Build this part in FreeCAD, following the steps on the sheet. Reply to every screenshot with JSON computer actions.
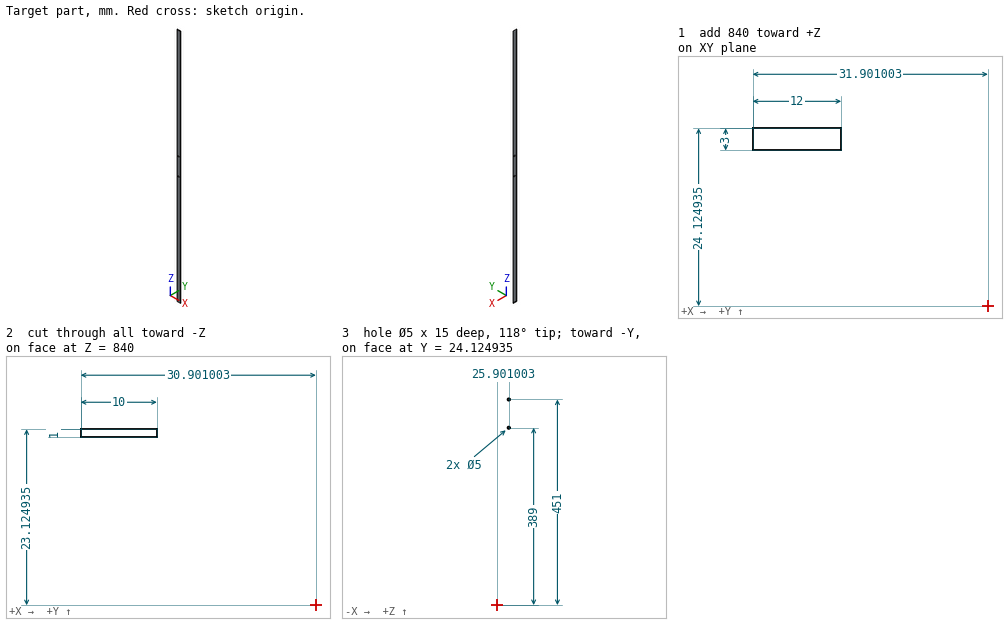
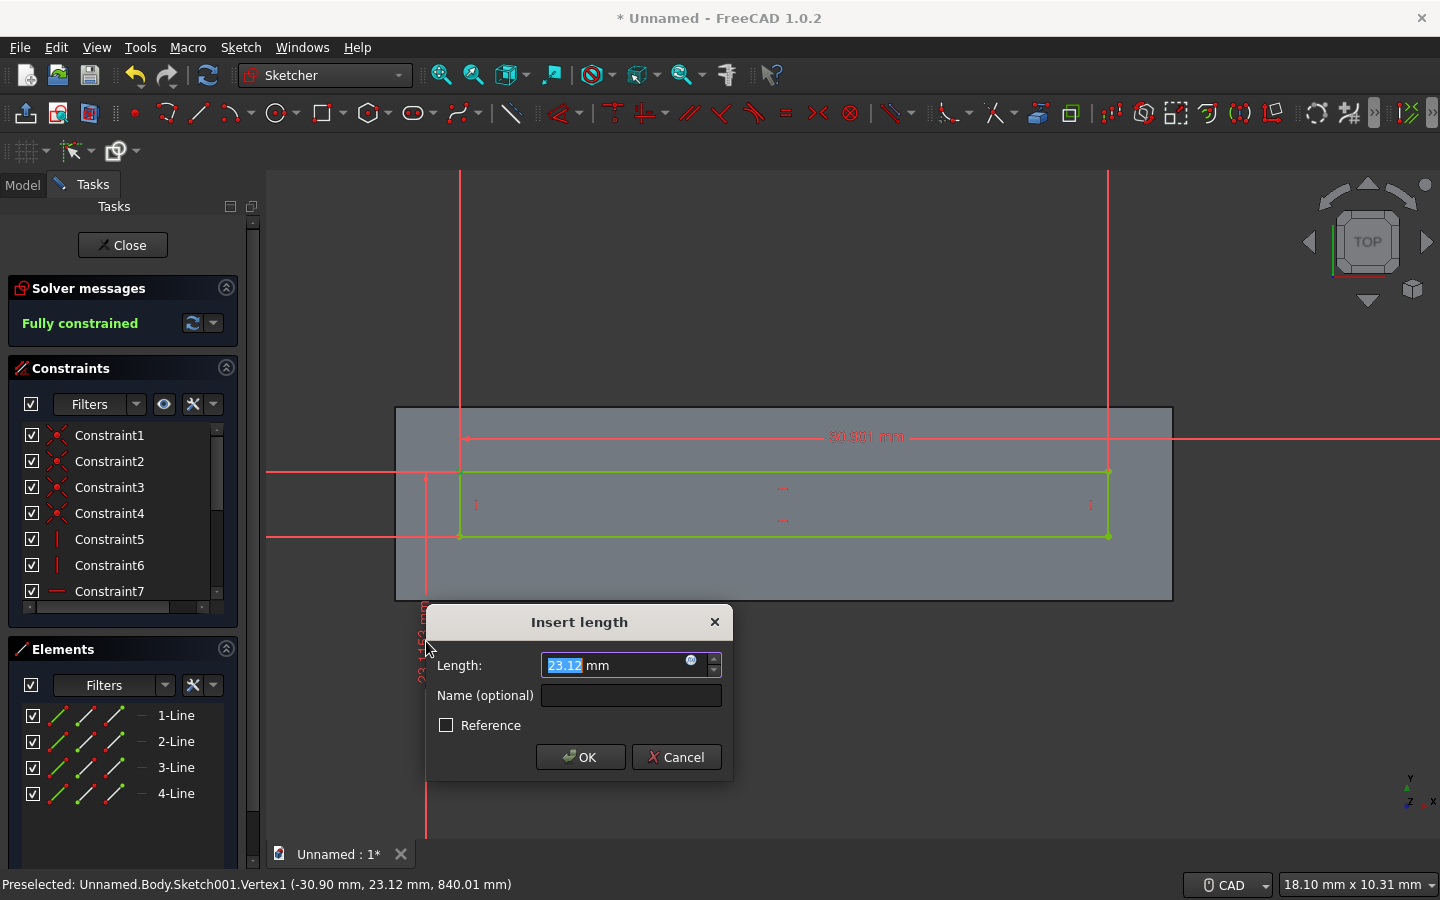
{"action": "type", "text": "23.124935"}
{"action": "key", "text": "Return"}
{"action": "key", "text": "Escape"}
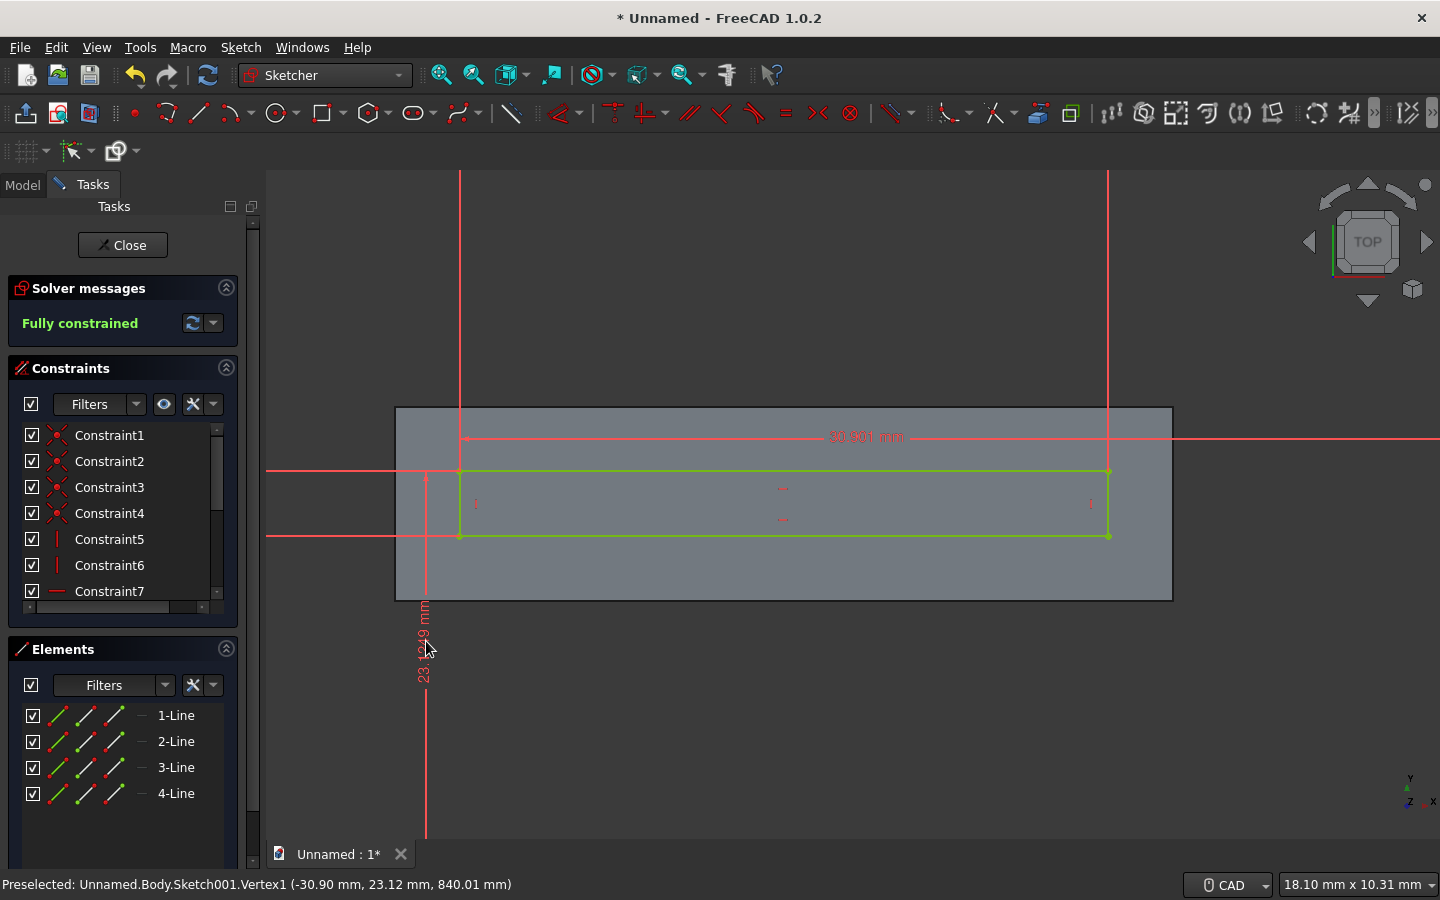
{"action": "left_click", "coordinate": [123, 245]}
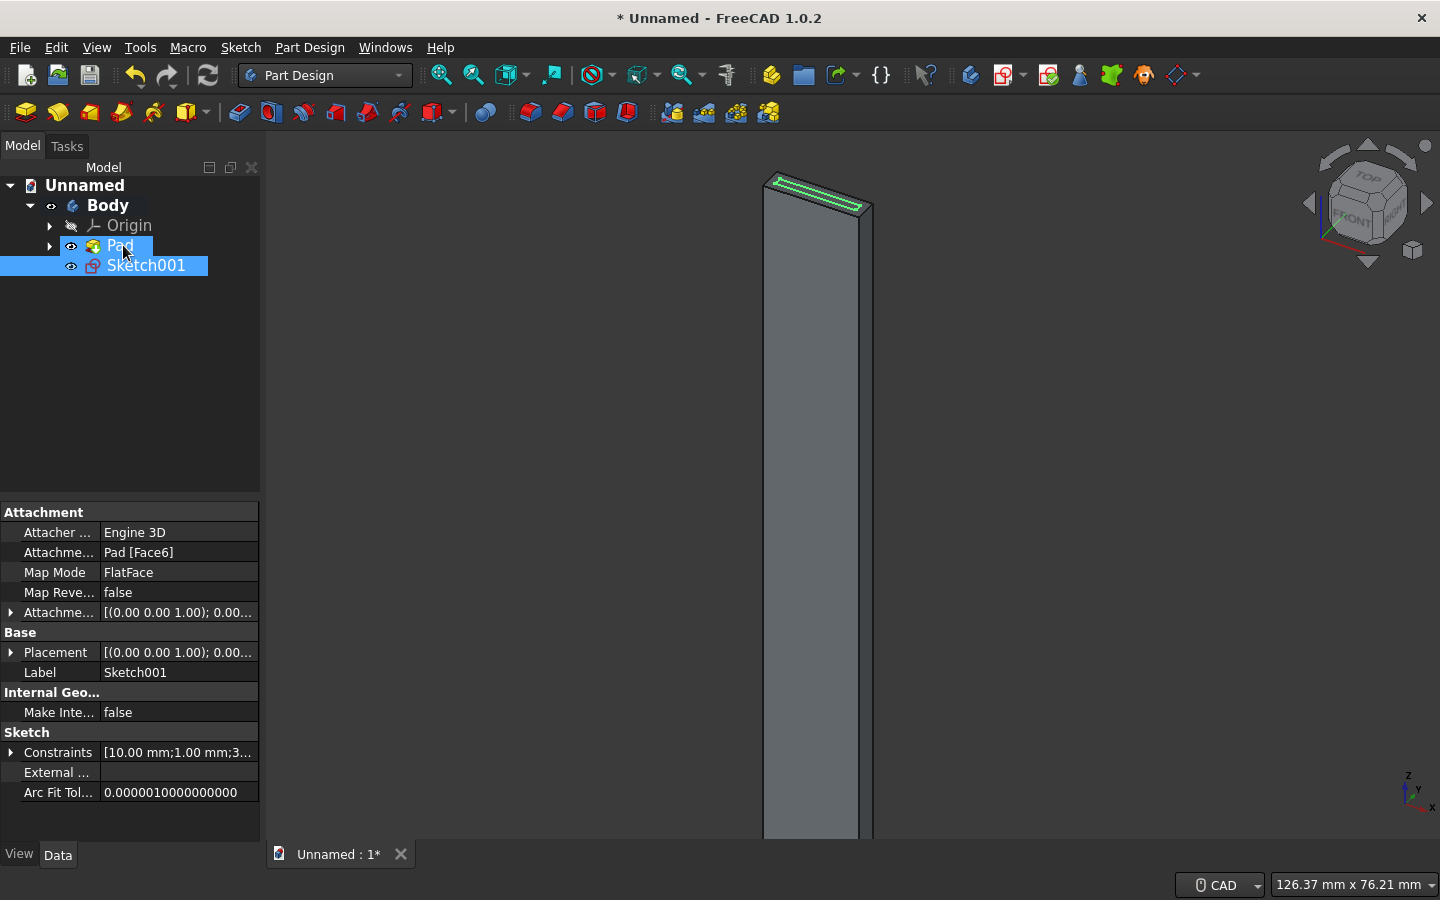
{"action": "left_click", "coordinate": [240, 112]}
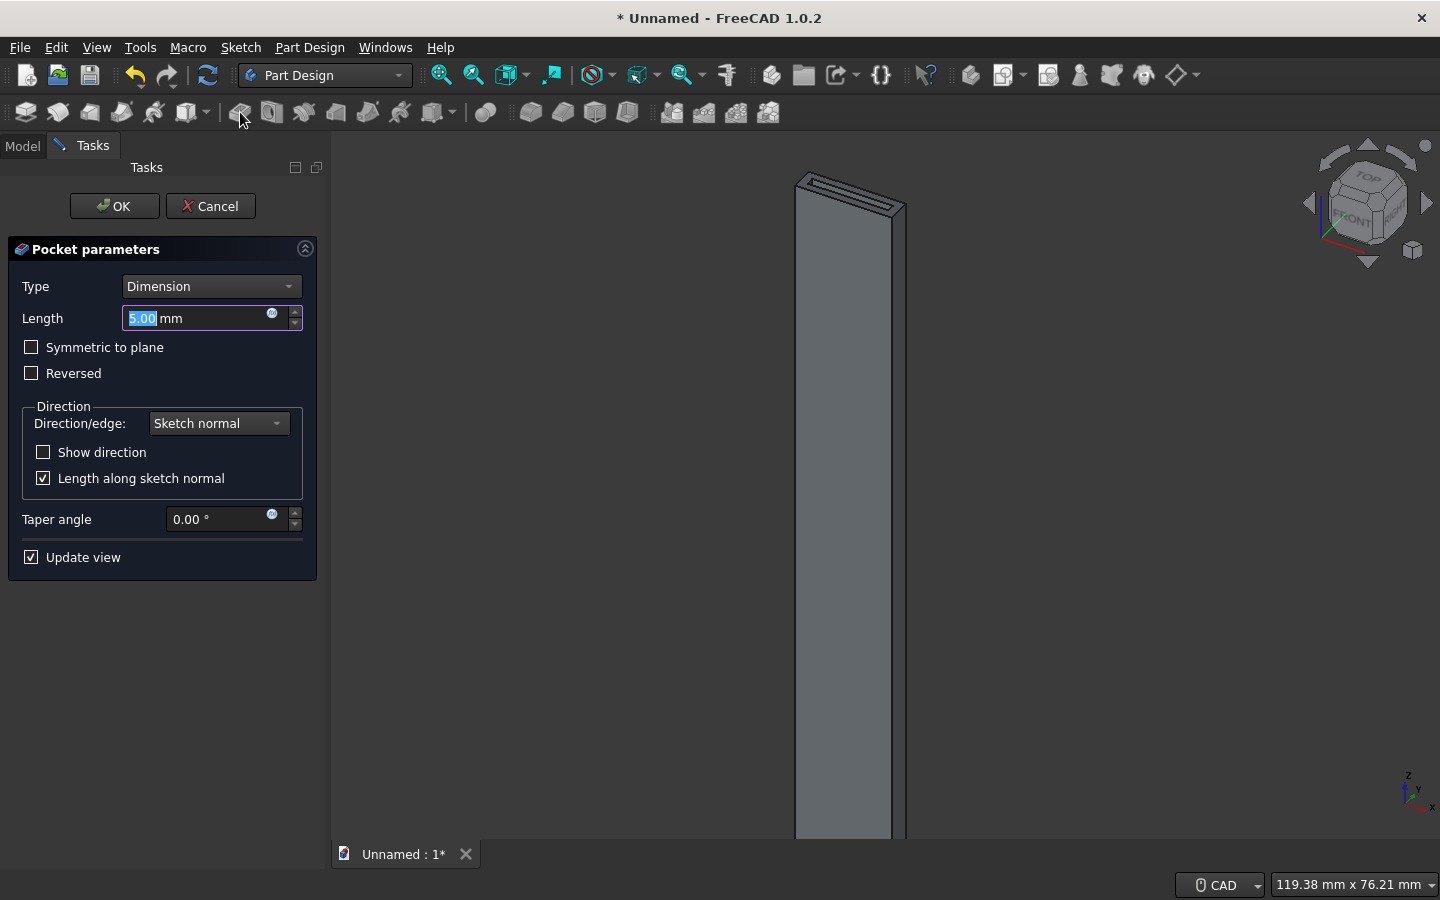
{"action": "left_click", "coordinate": [212, 286]}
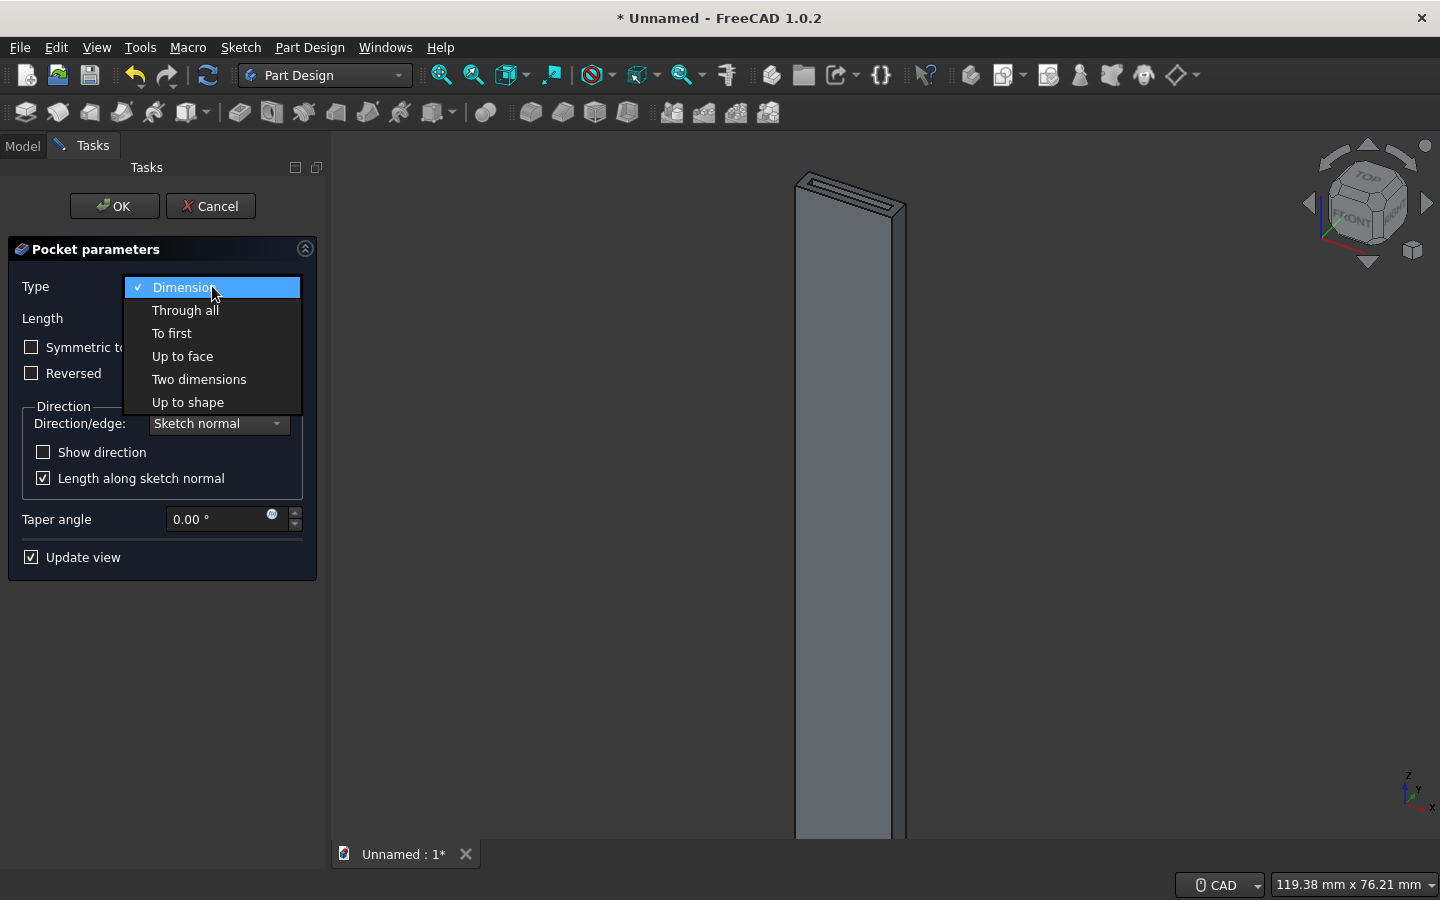
{"action": "left_click", "coordinate": [212, 310]}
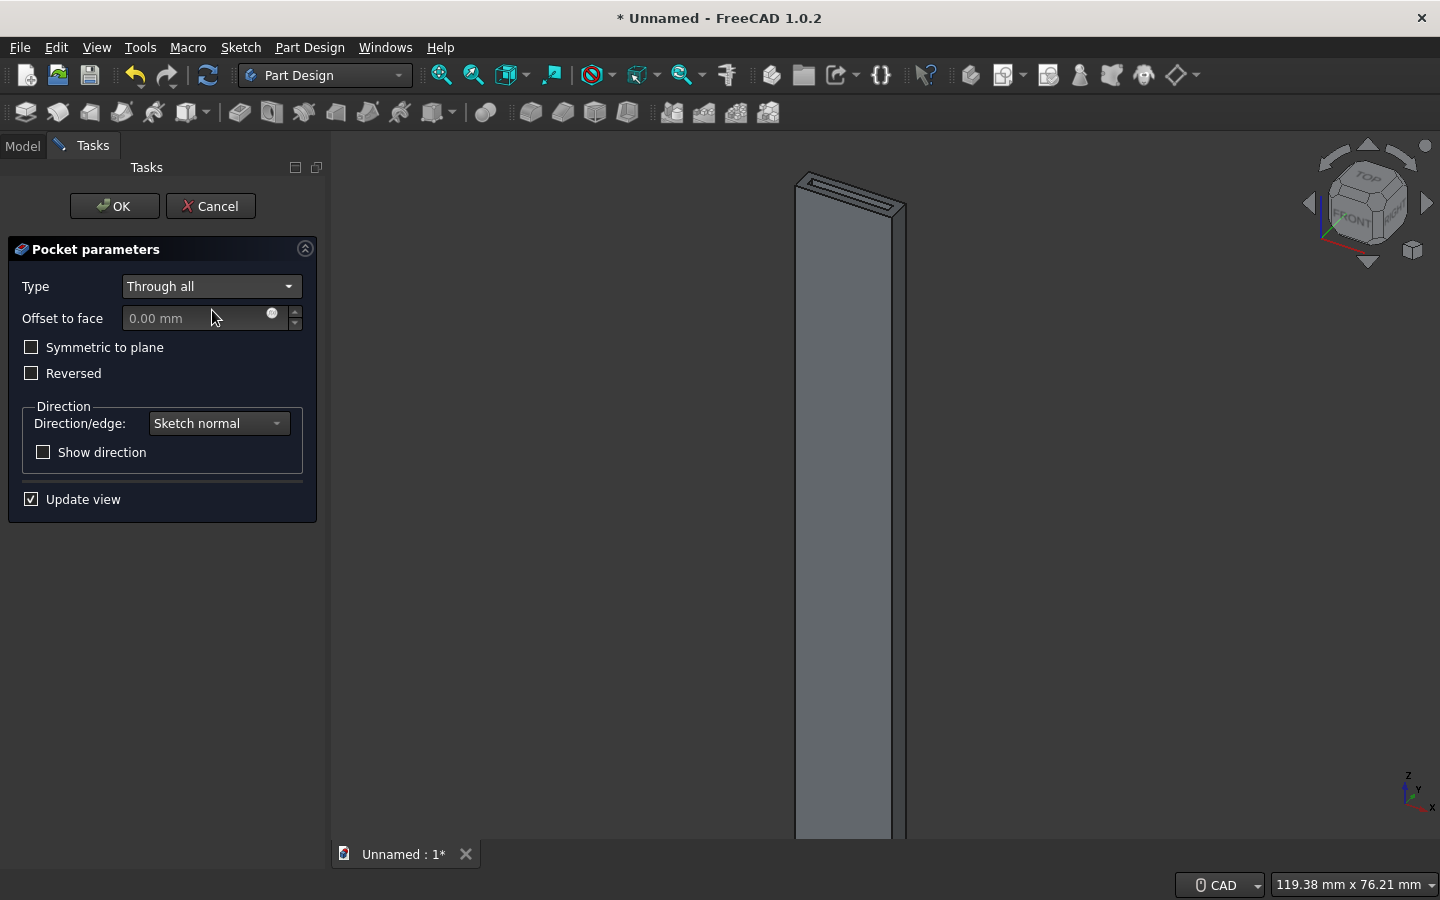
{"action": "left_click", "coordinate": [115, 206]}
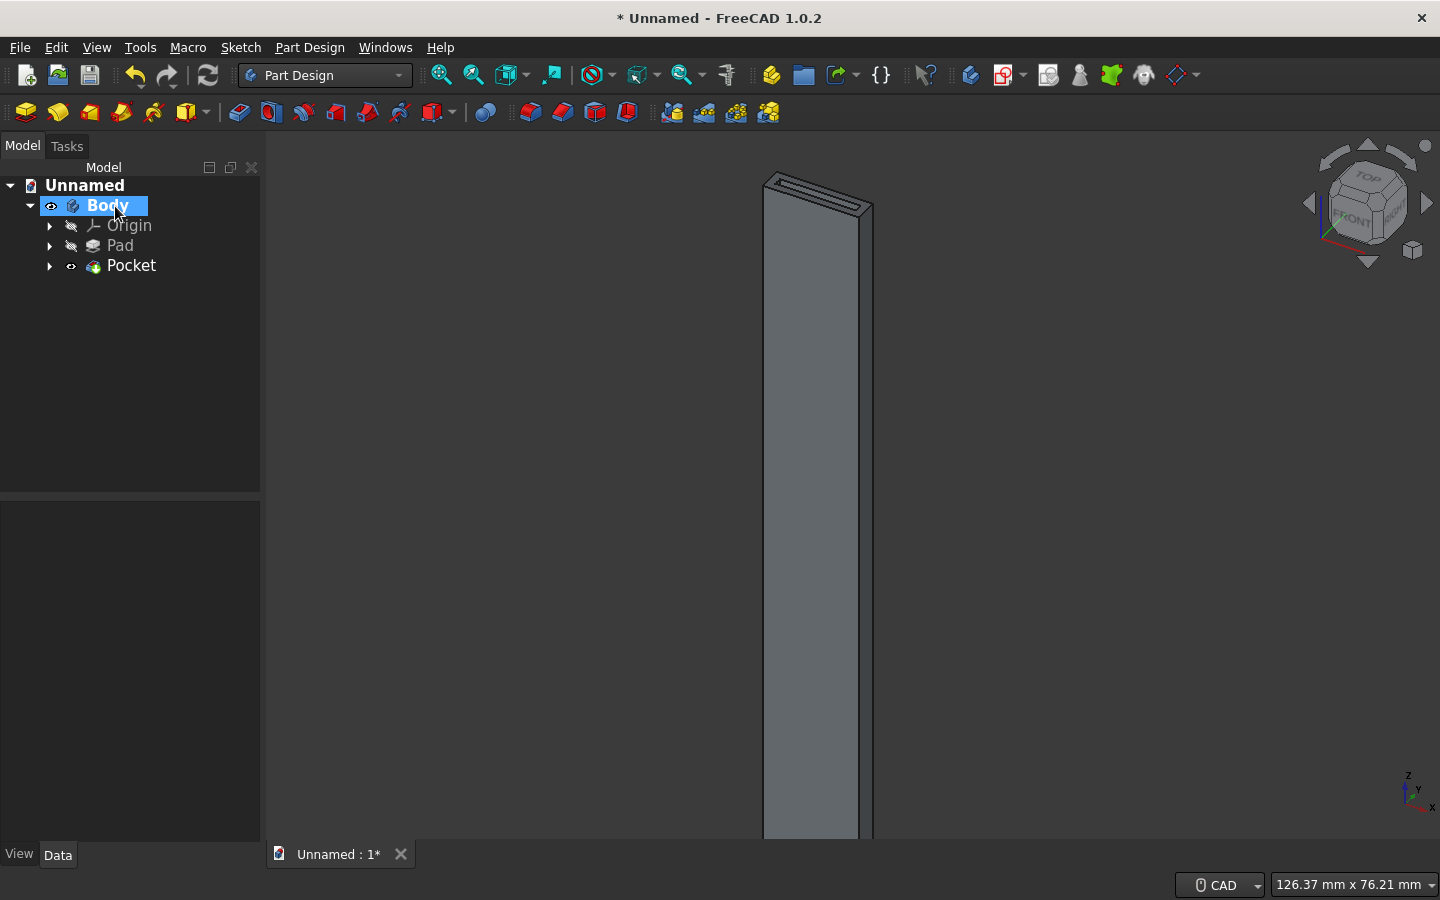
{"action": "key", "text": "v f"}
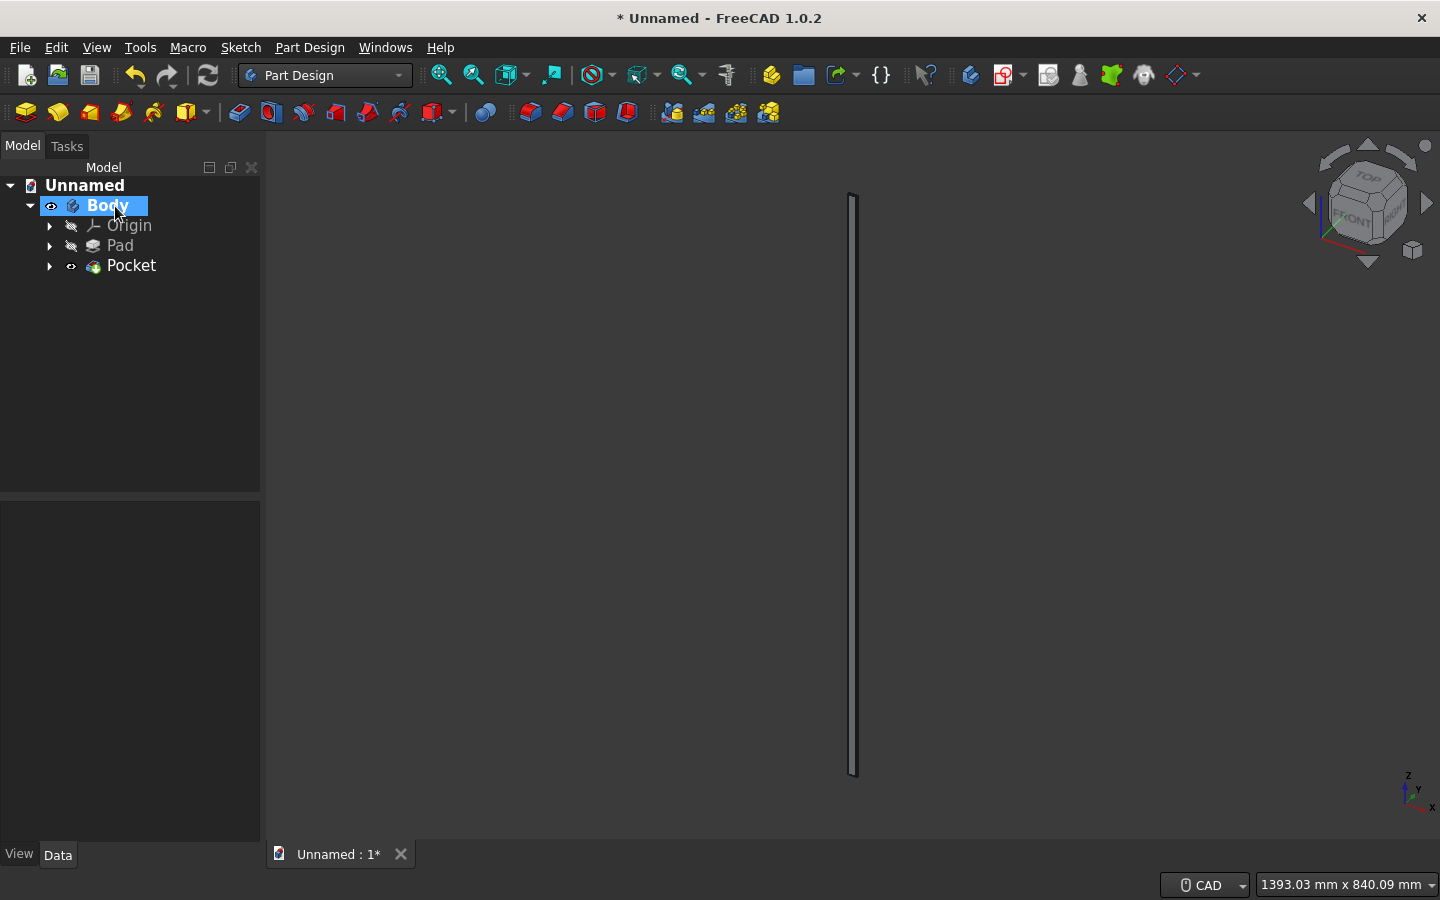
{"action": "key", "text": "4"}